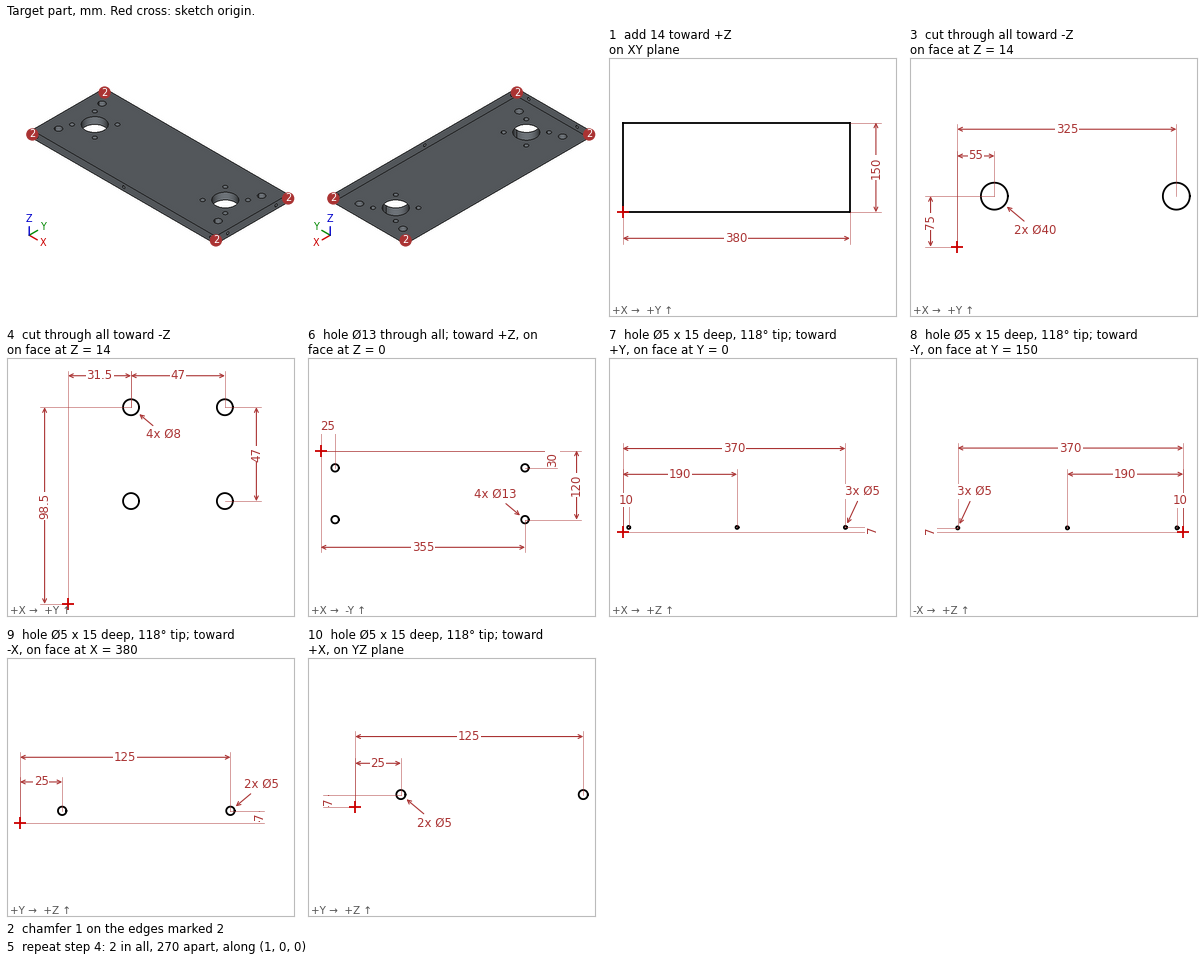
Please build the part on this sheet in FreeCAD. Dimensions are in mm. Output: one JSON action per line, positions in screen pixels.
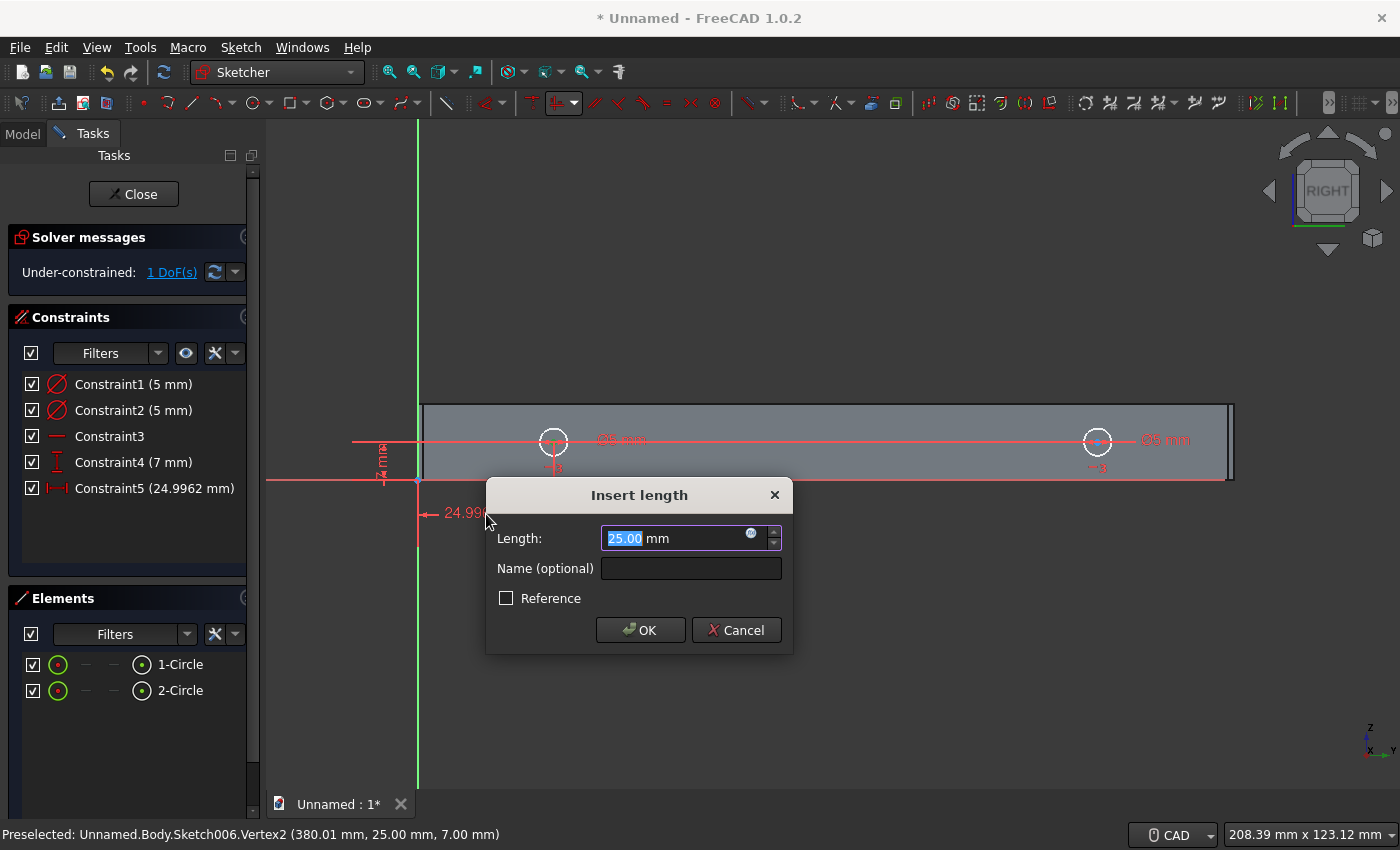
{"action": "type", "text": "25"}
{"action": "key", "text": "Return"}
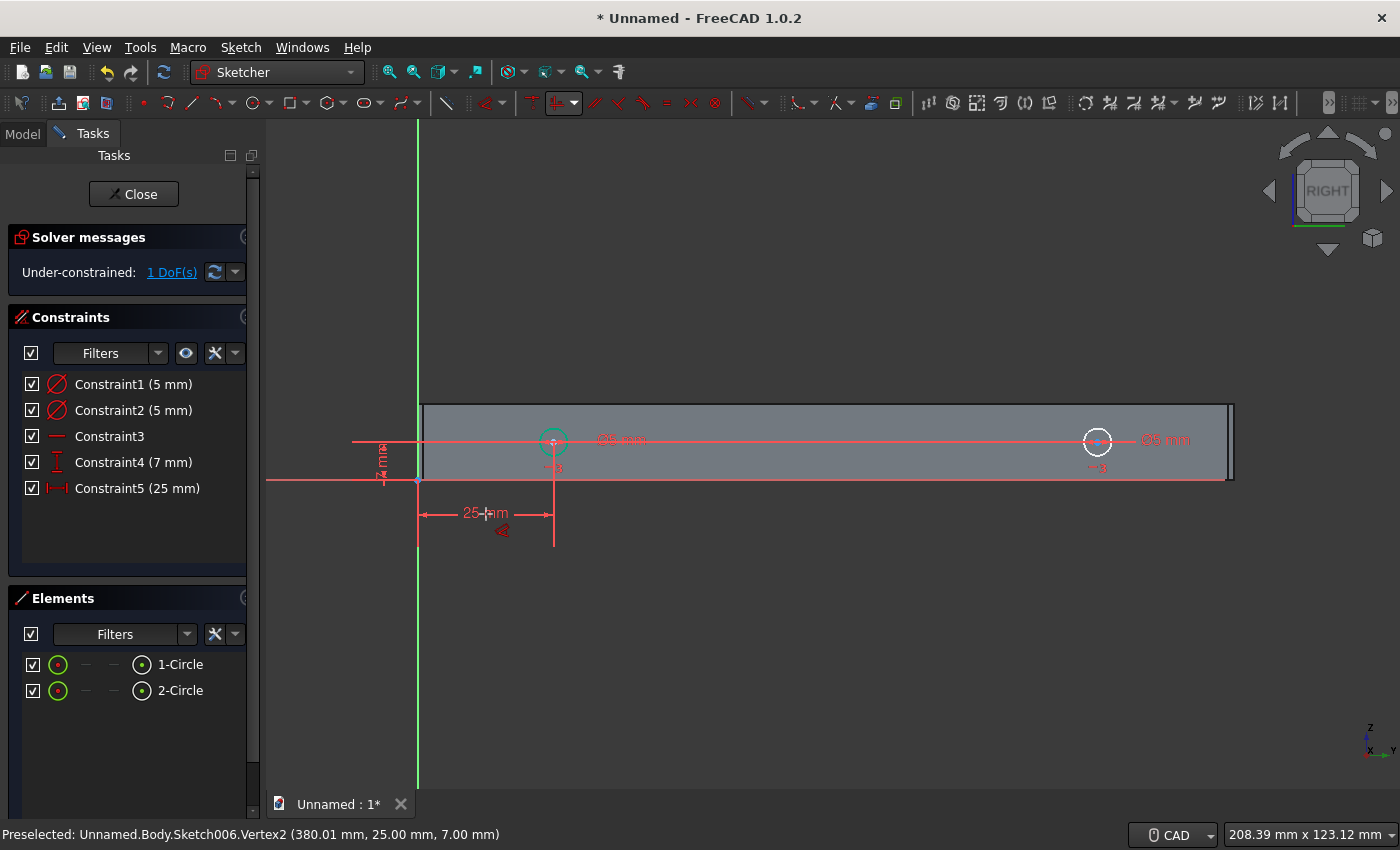
{"action": "left_click", "coordinate": [1098, 442]}
{"action": "left_click", "coordinate": [758, 514]}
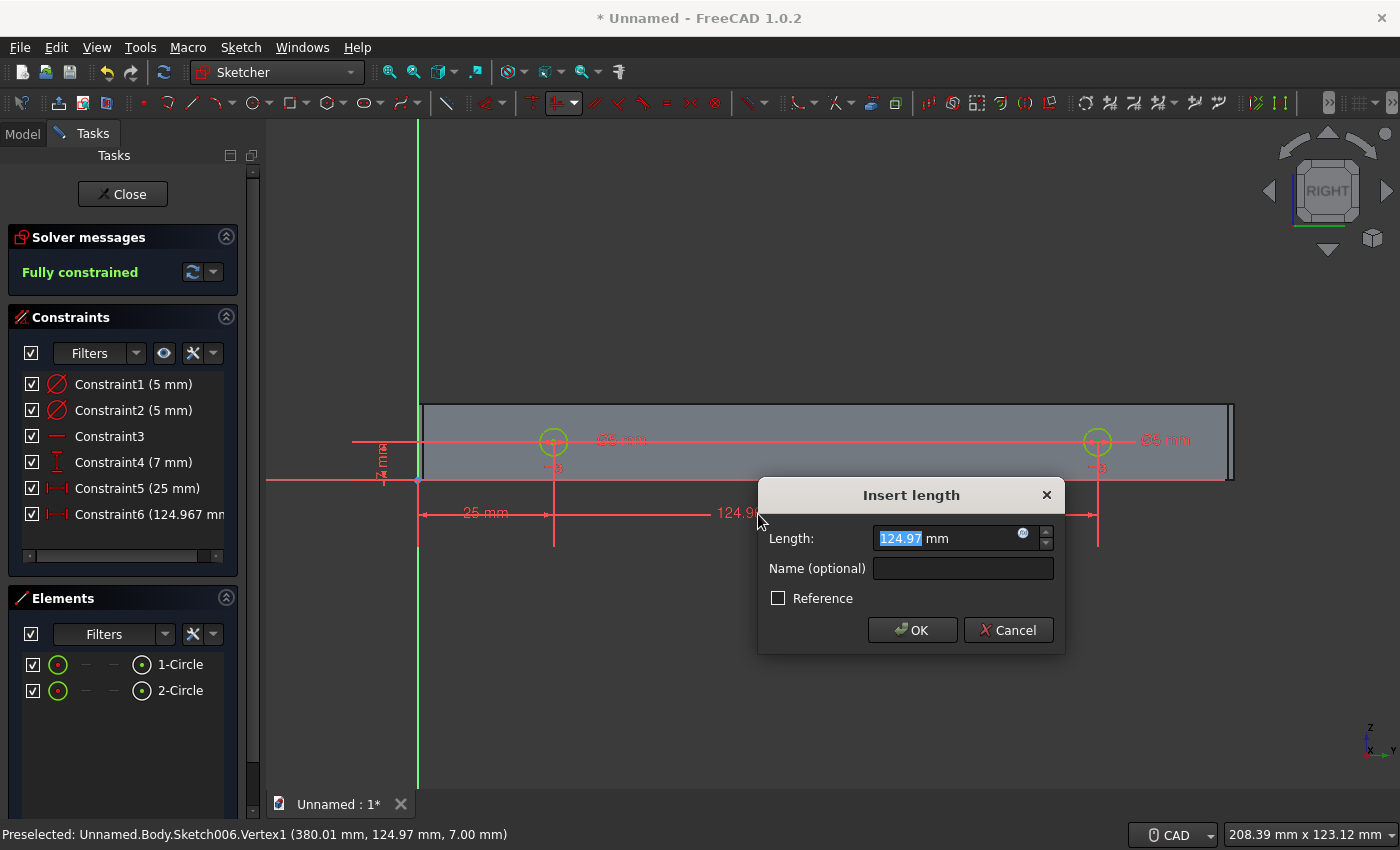
{"action": "type", "text": "125"}
{"action": "key", "text": "Return"}
{"action": "key", "text": "Escape"}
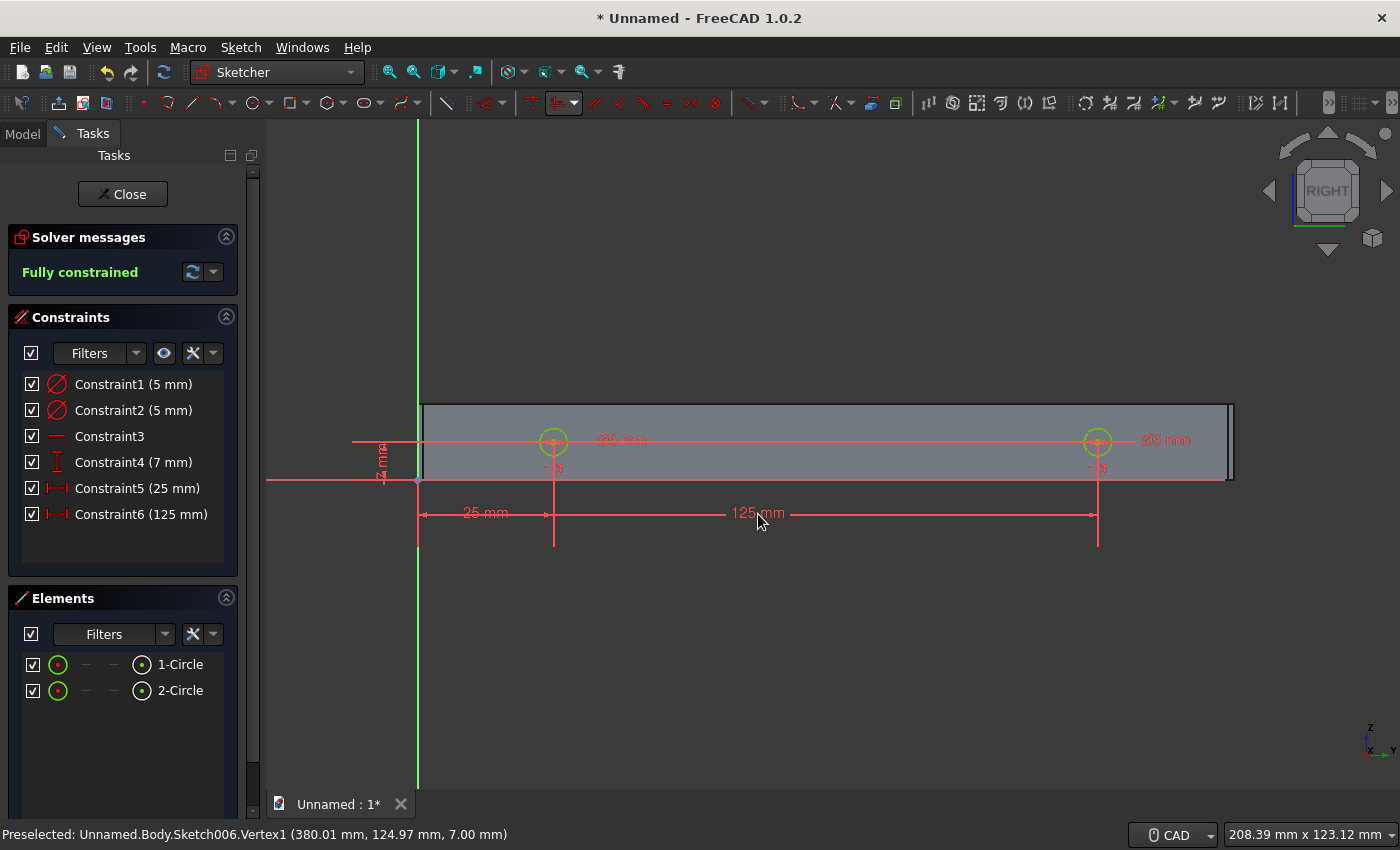
{"action": "left_click", "coordinate": [123, 194]}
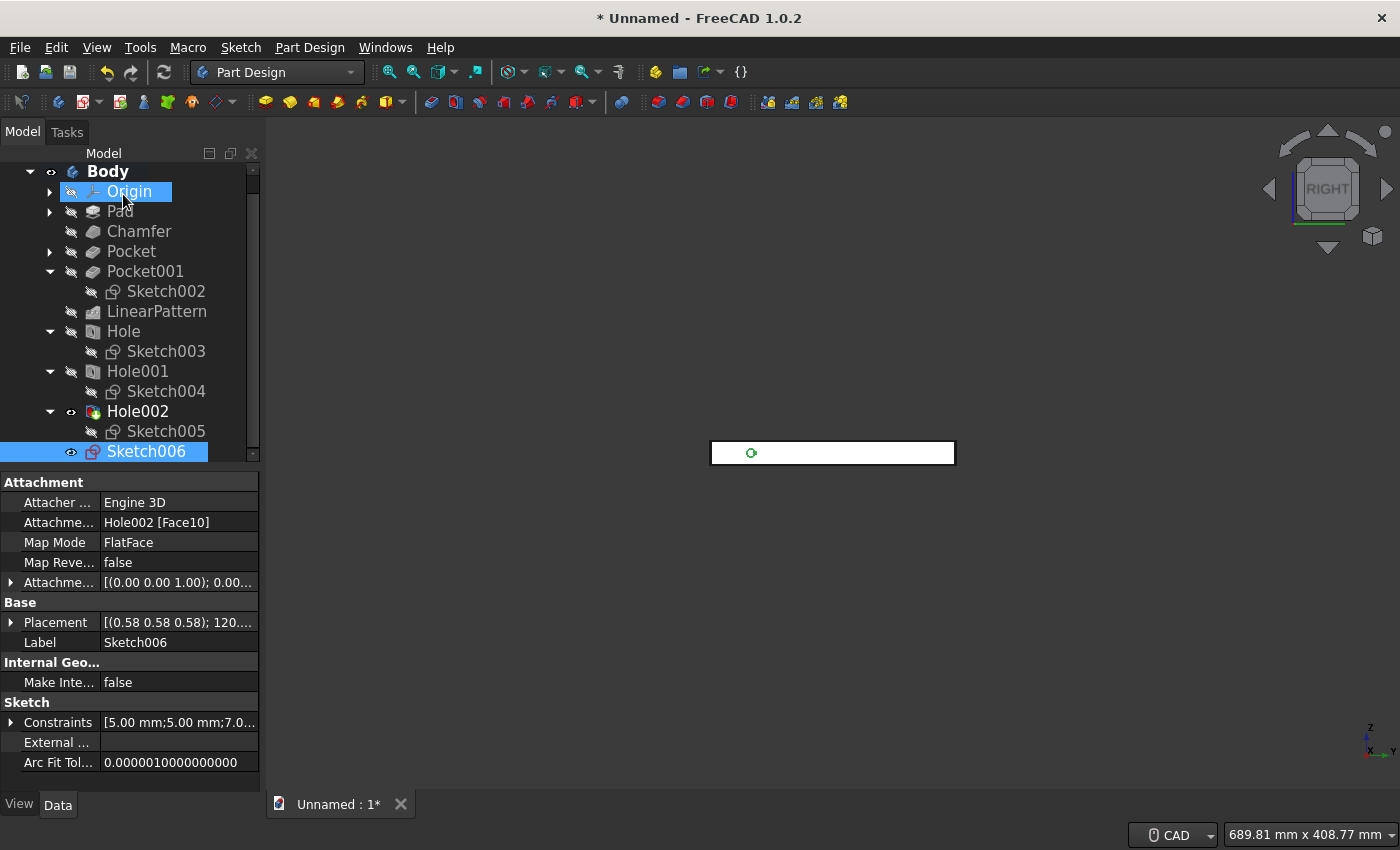
{"action": "left_click", "coordinate": [456, 102]}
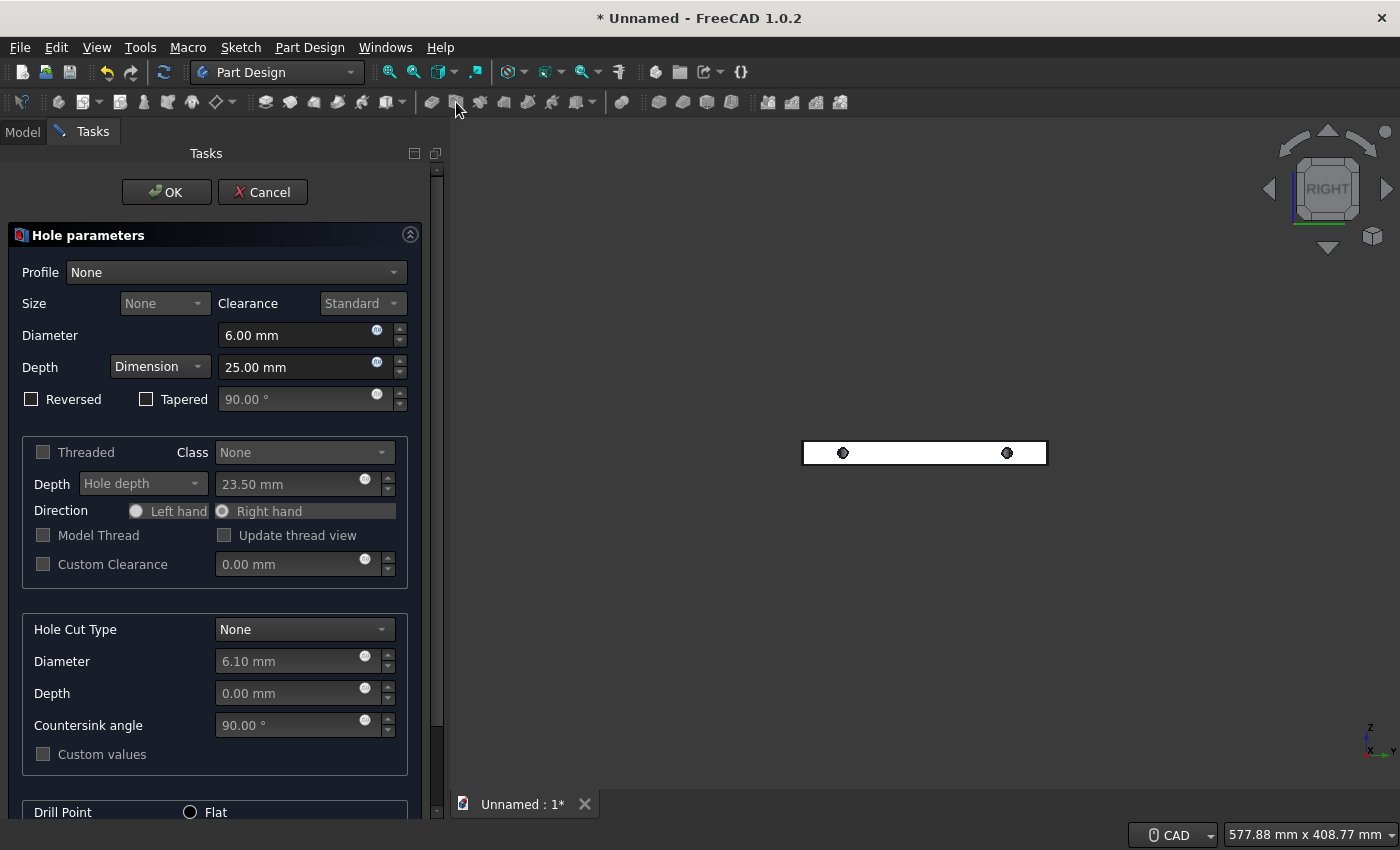
{"action": "triple_click", "coordinate": [305, 335]}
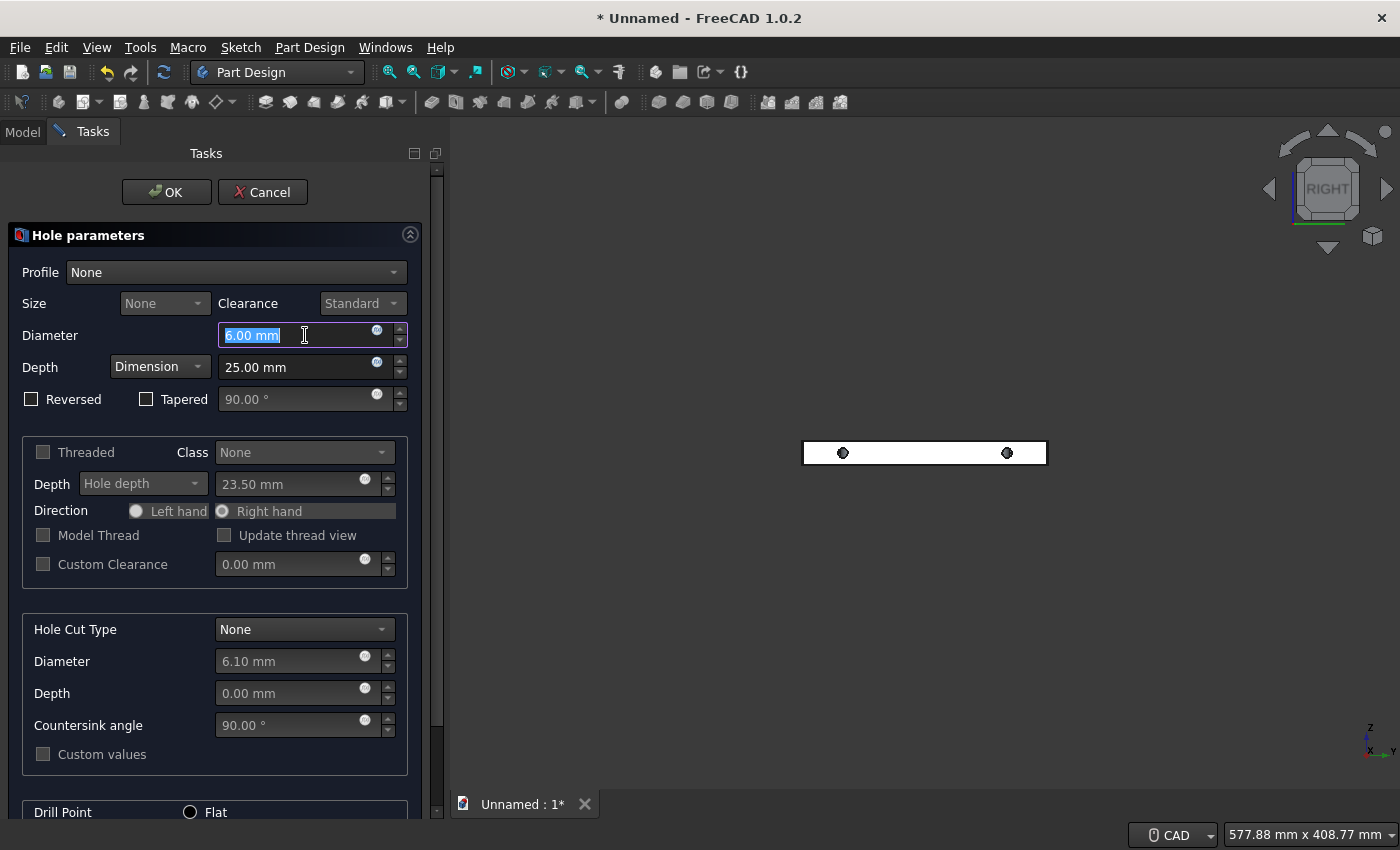
{"action": "type", "text": "5"}
{"action": "key", "text": "Tab"}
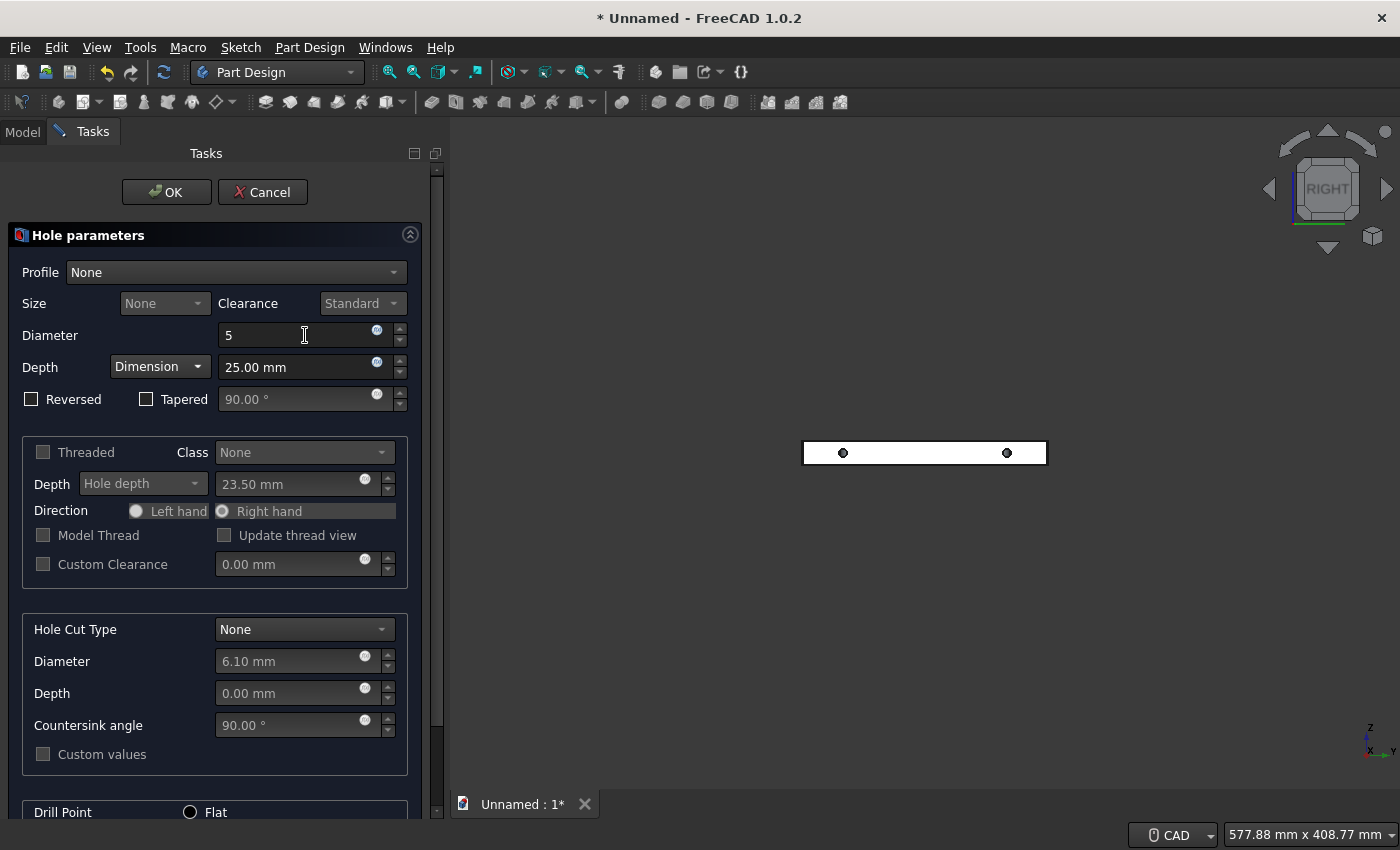
{"action": "triple_click", "coordinate": [305, 367]}